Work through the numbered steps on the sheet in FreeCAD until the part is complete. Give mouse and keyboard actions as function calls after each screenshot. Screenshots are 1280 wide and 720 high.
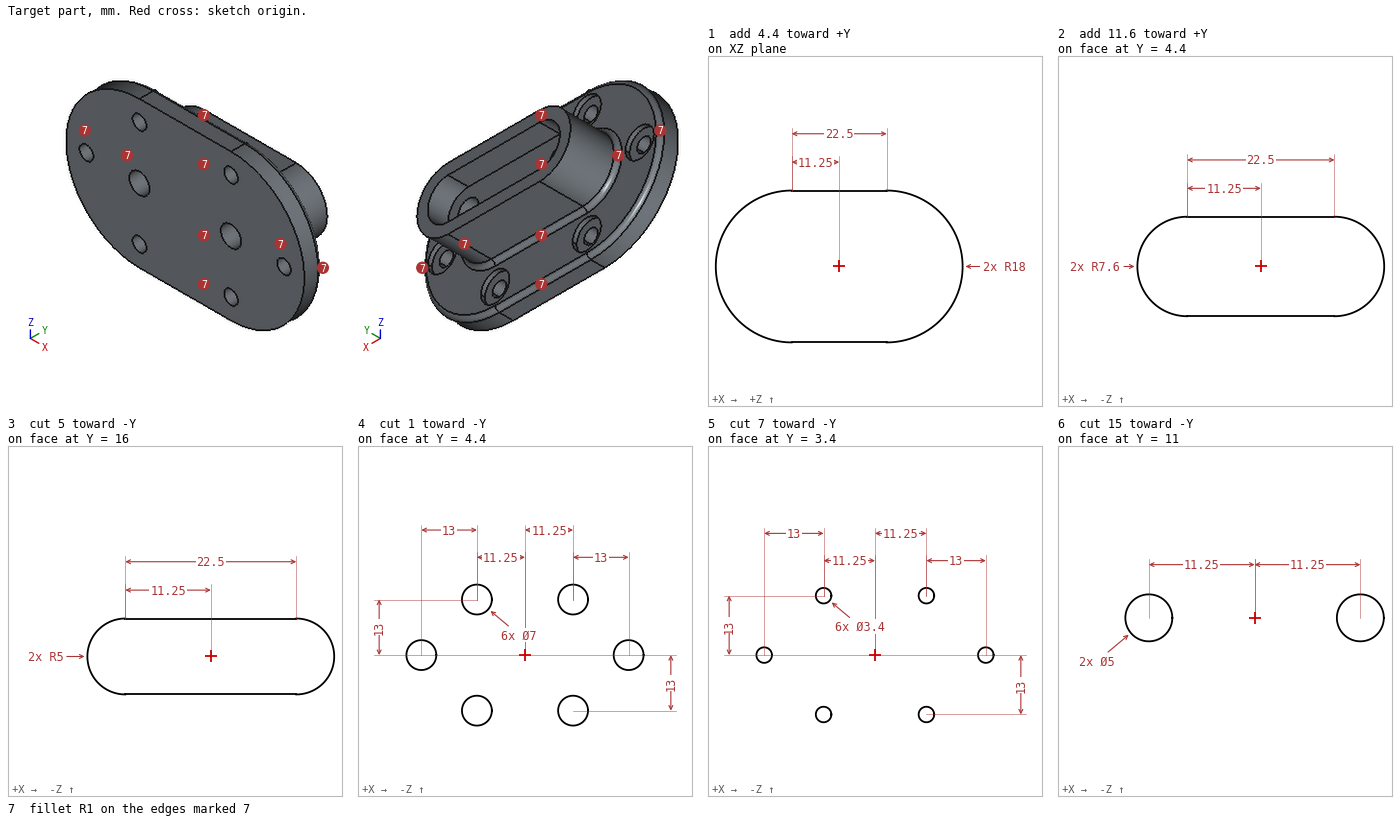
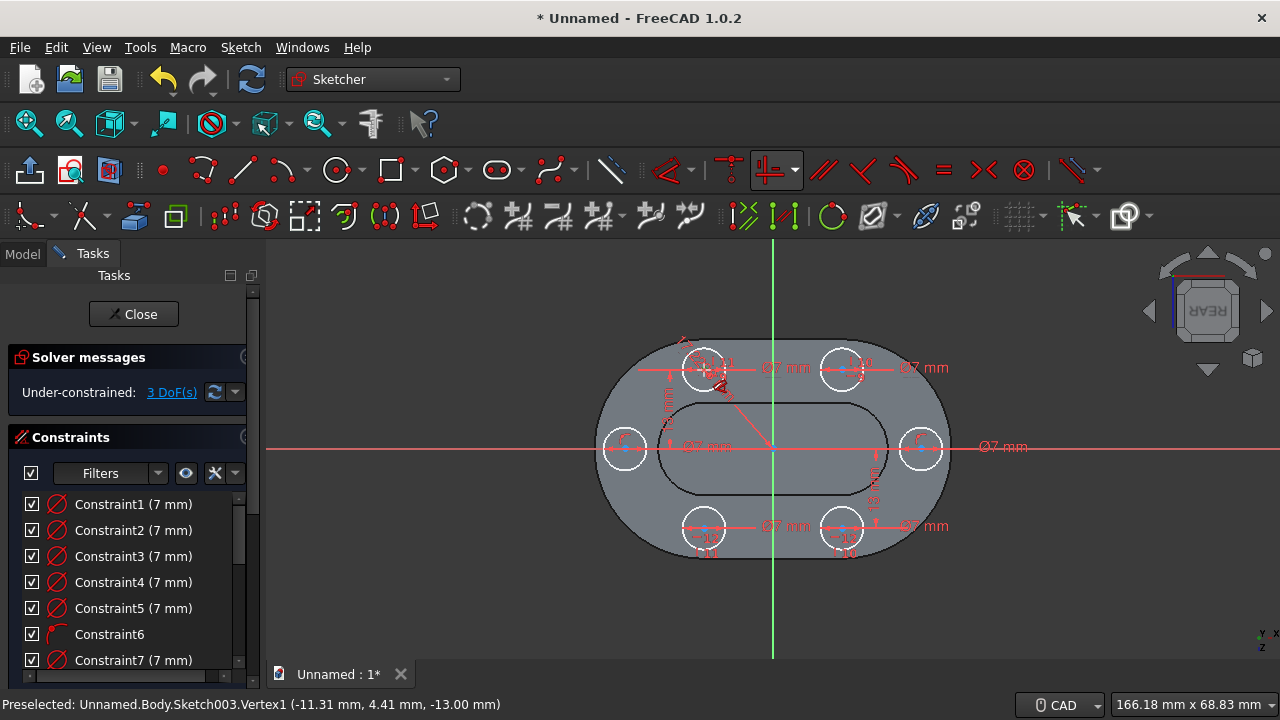
click(625, 449)
click(665, 336)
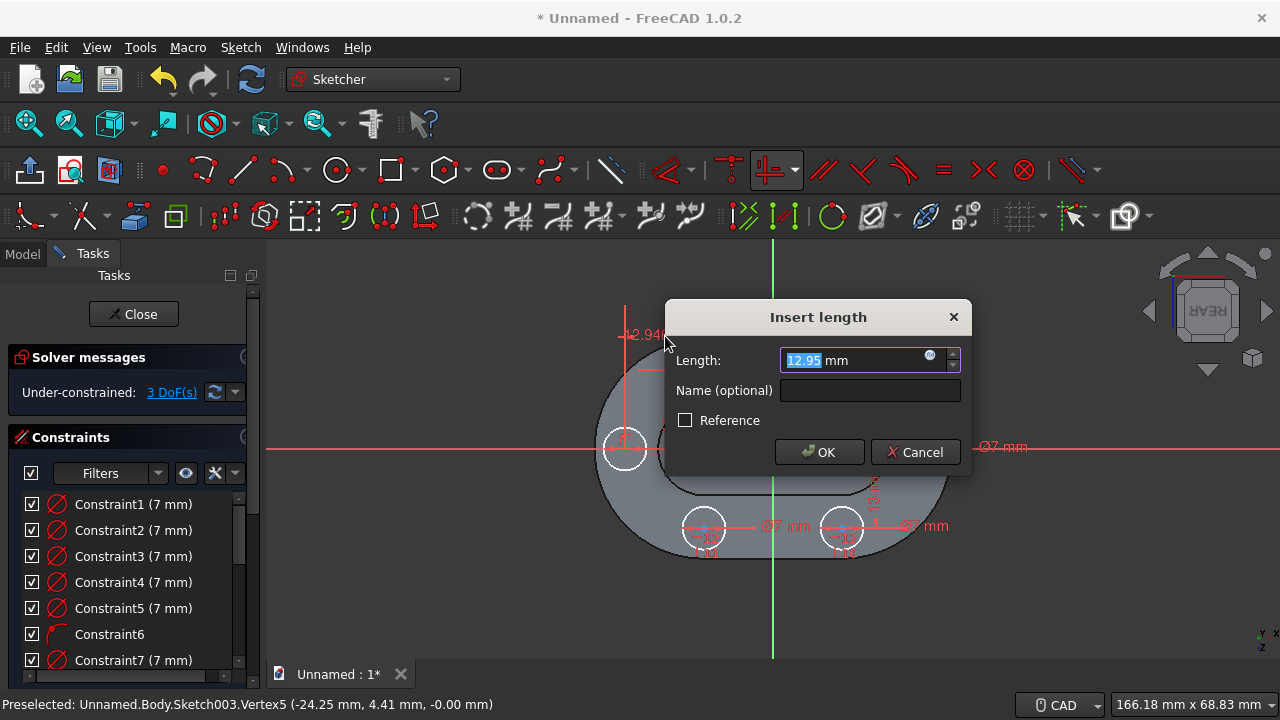
text(13)
key(Return)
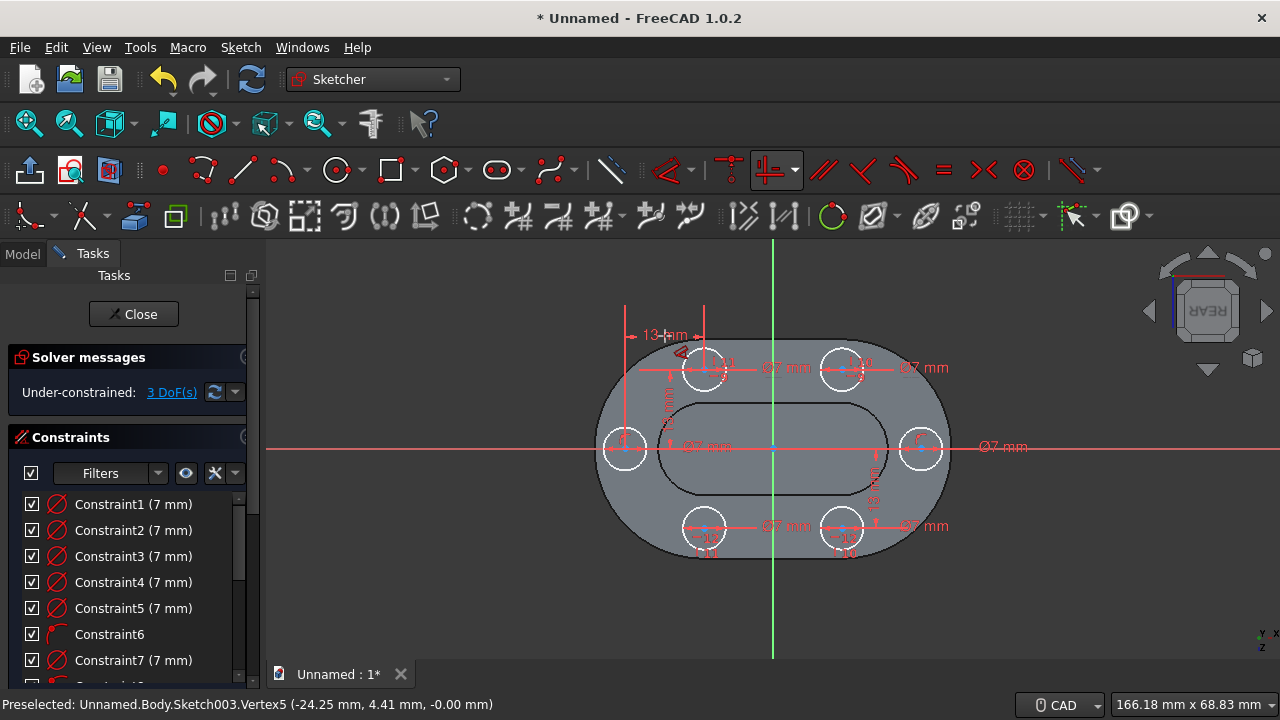
click(842, 370)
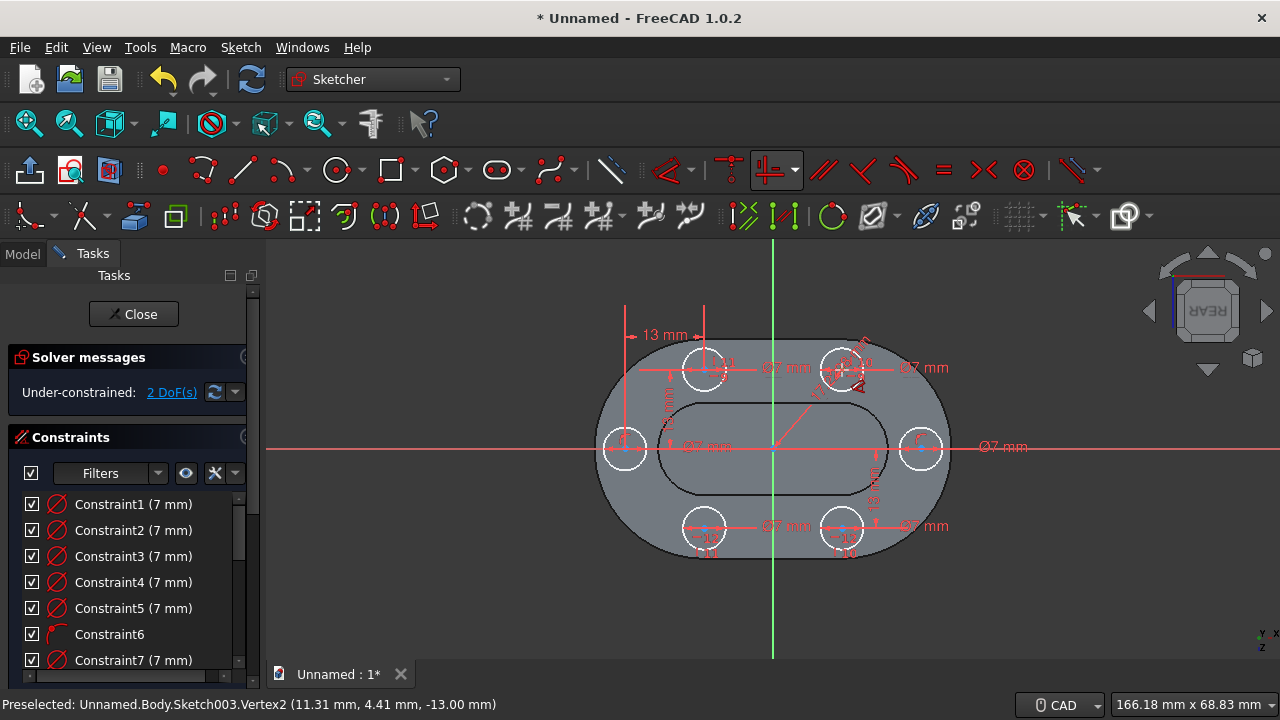
click(921, 449)
click(882, 336)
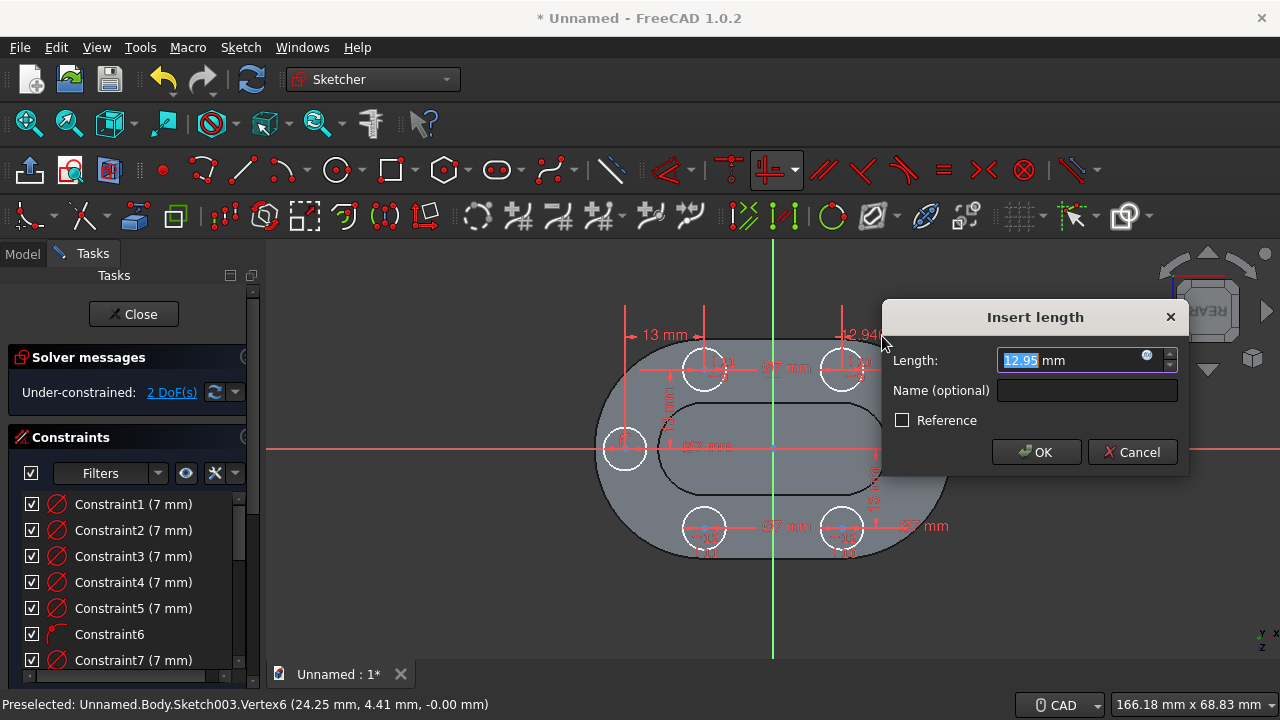
text(13)
key(Return)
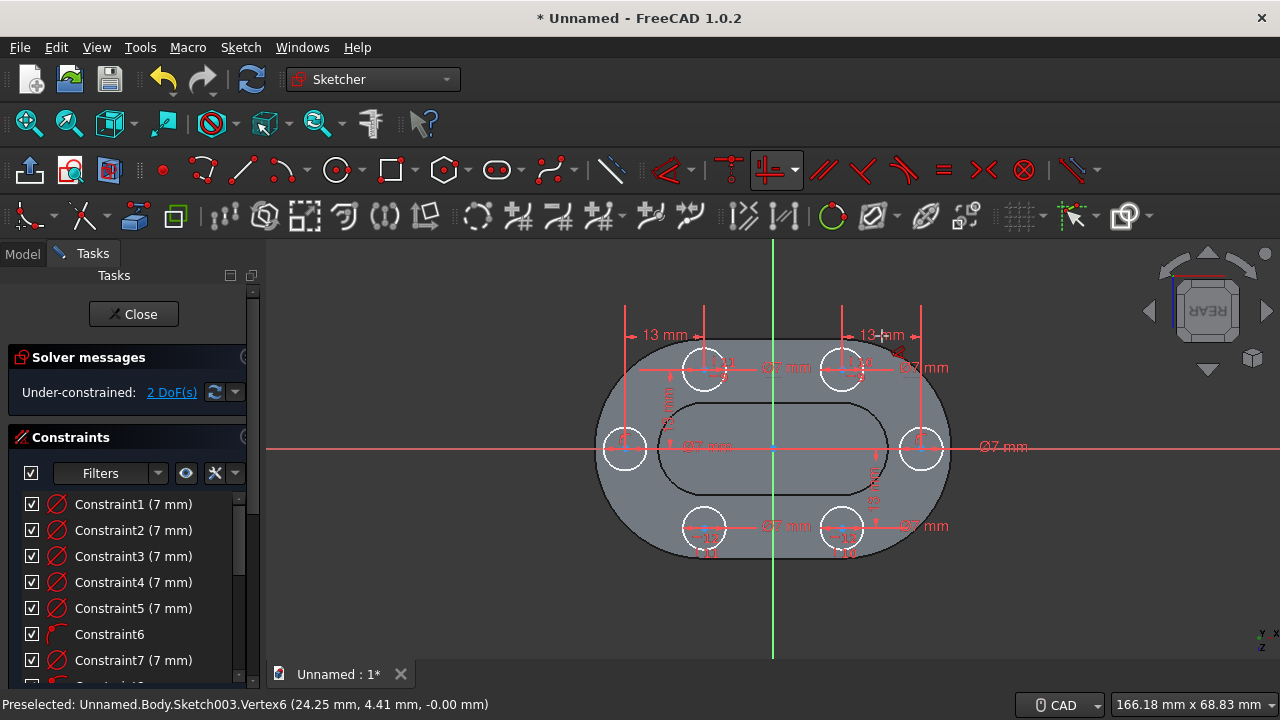
click(704, 370)
click(739, 336)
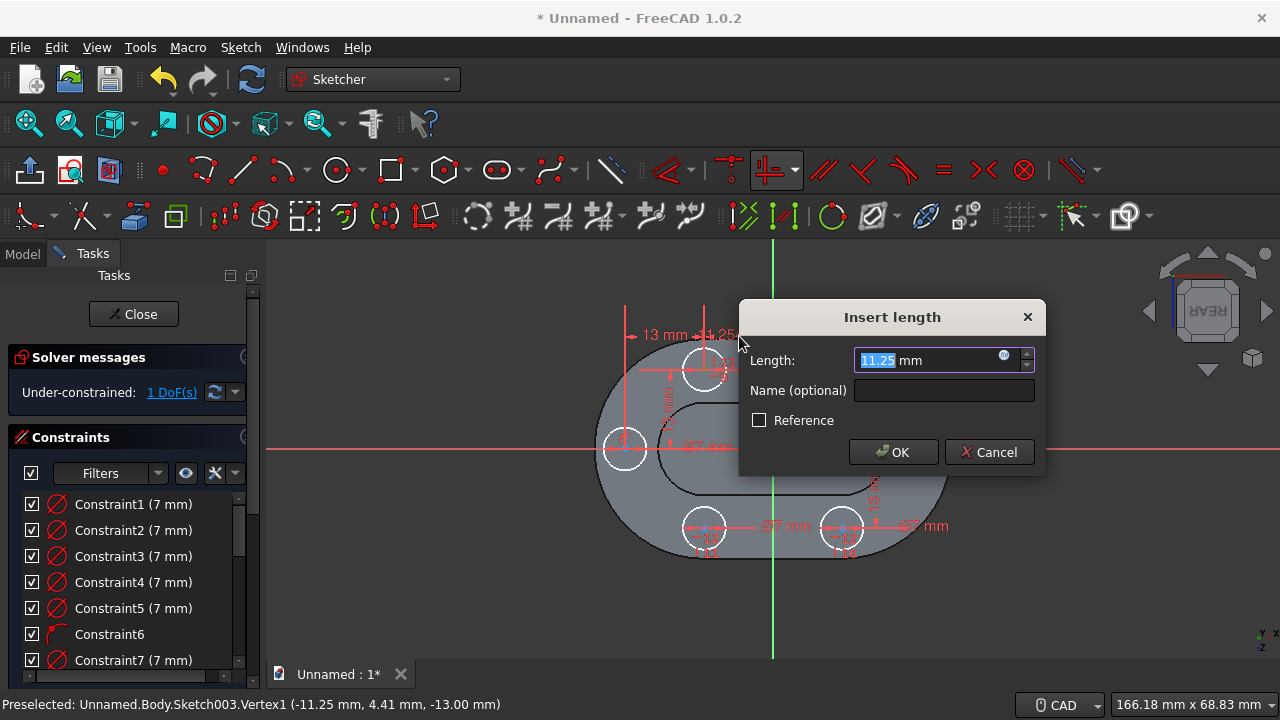
text(11.25)
key(Return)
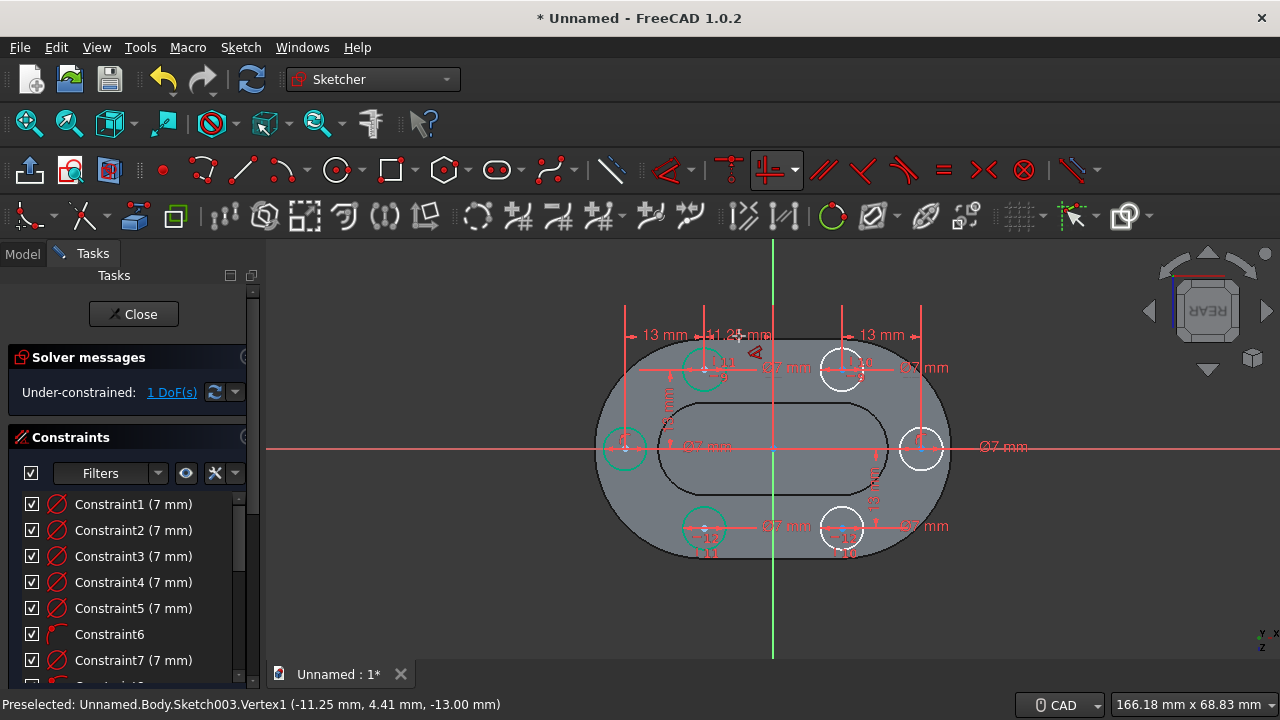
click(842, 370)
click(792, 483)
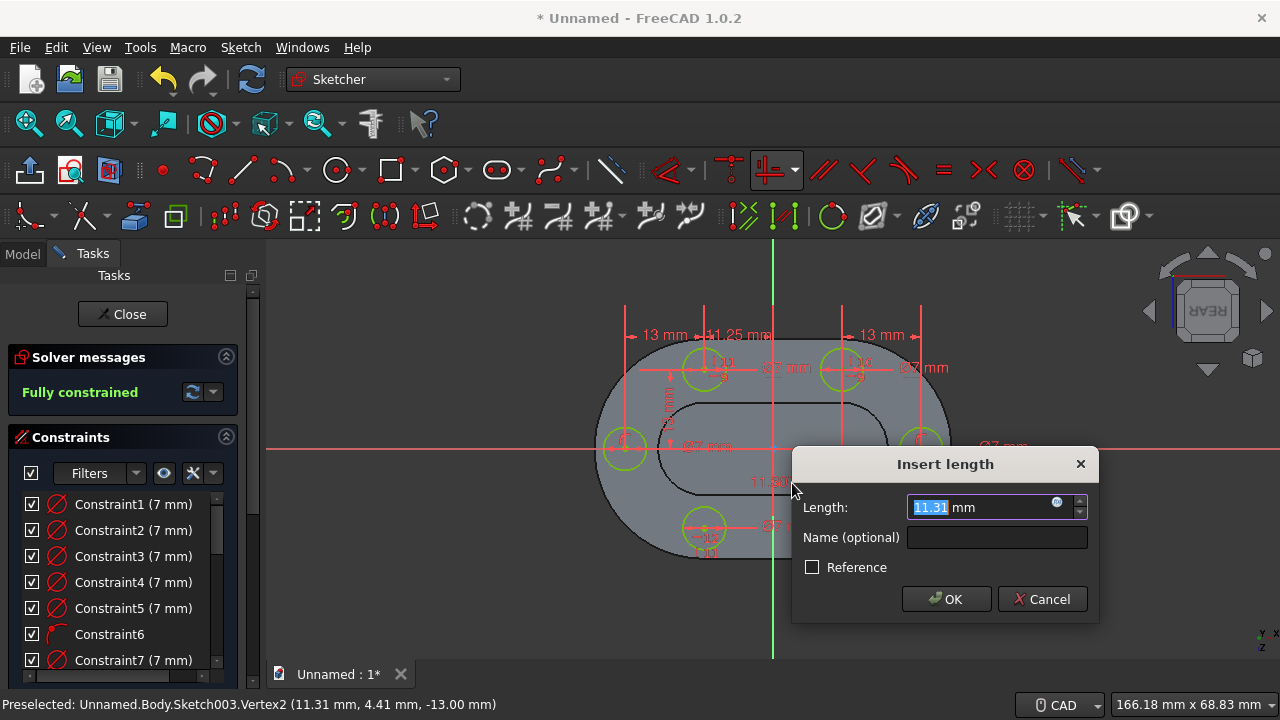
text(11.25)
key(Return)
key(Escape)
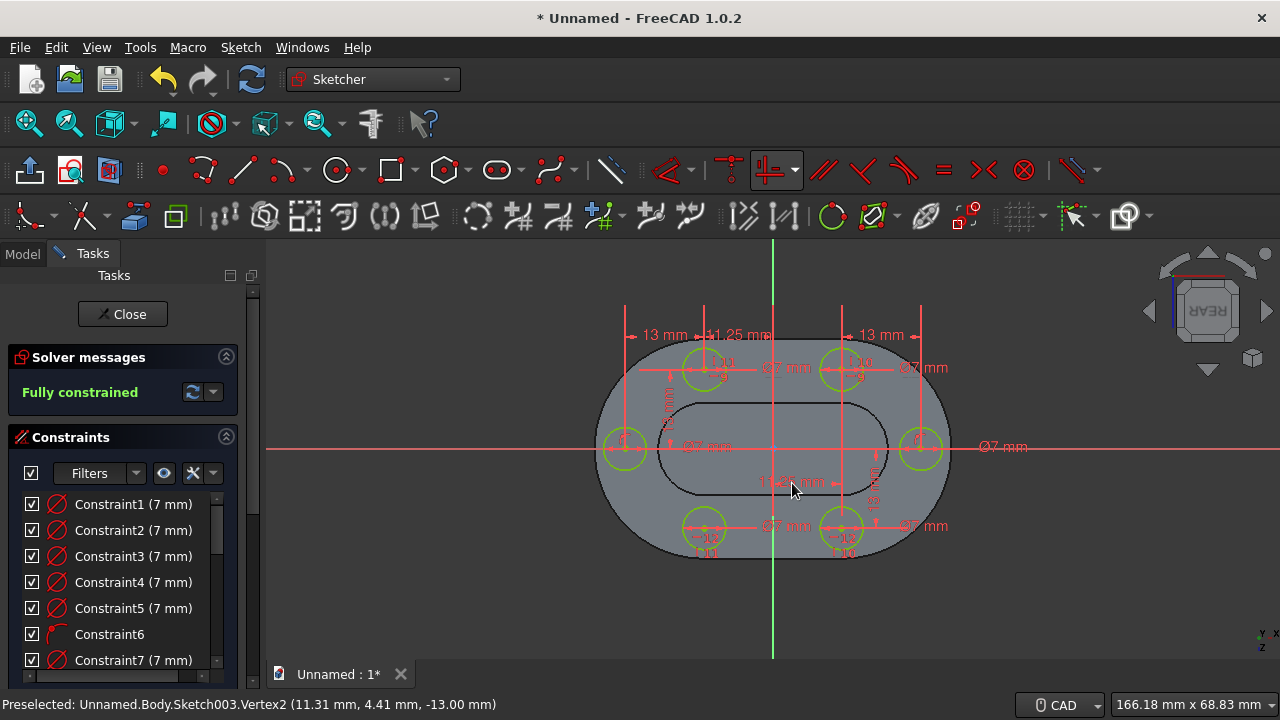
click(123, 314)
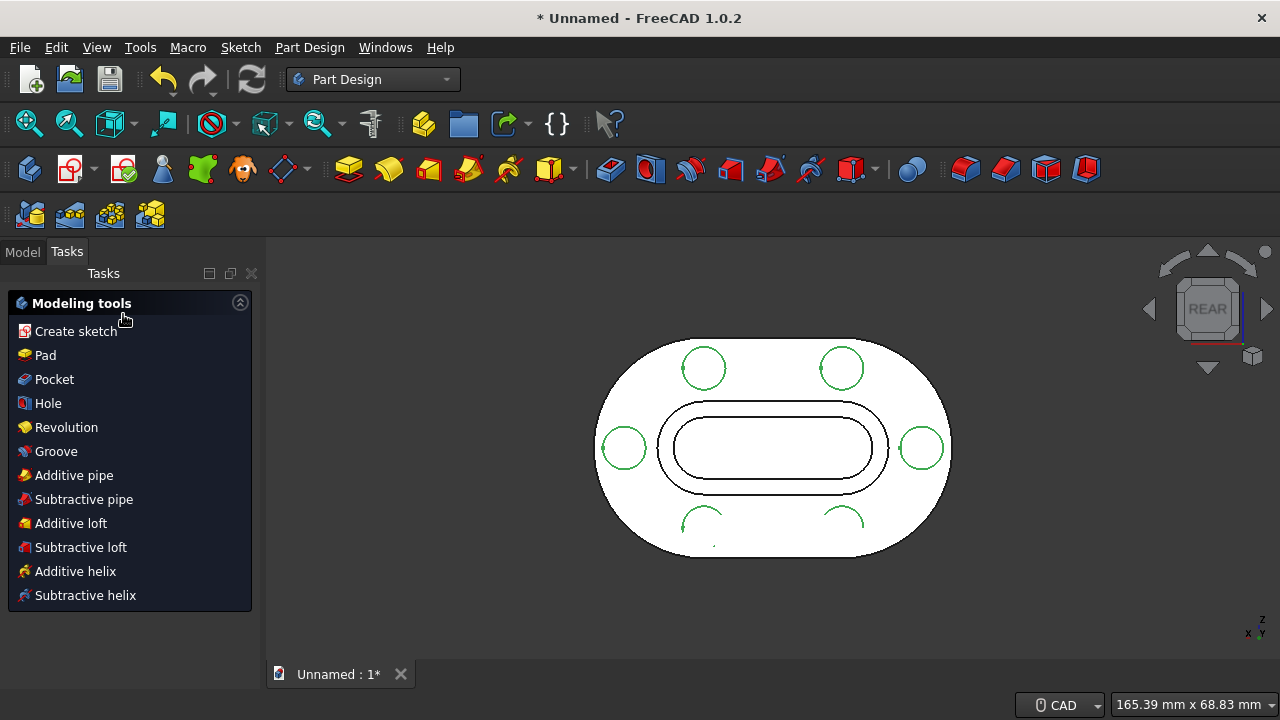
click(612, 170)